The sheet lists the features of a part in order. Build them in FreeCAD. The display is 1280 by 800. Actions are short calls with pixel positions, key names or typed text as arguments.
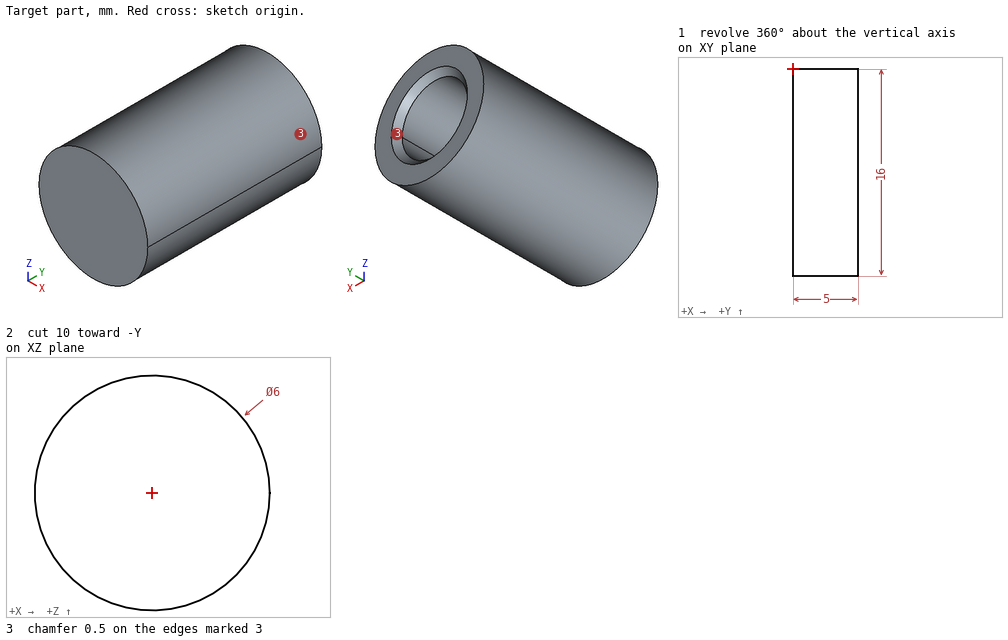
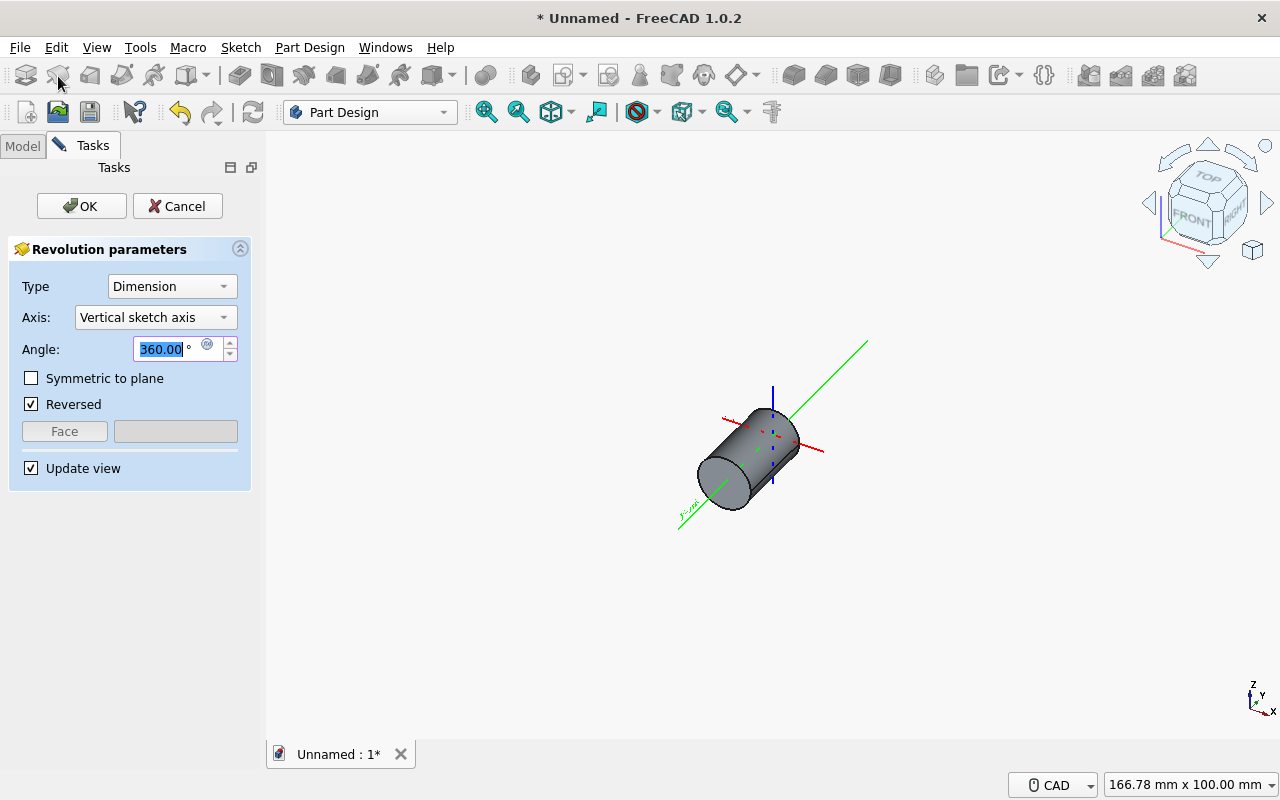
click(82, 206)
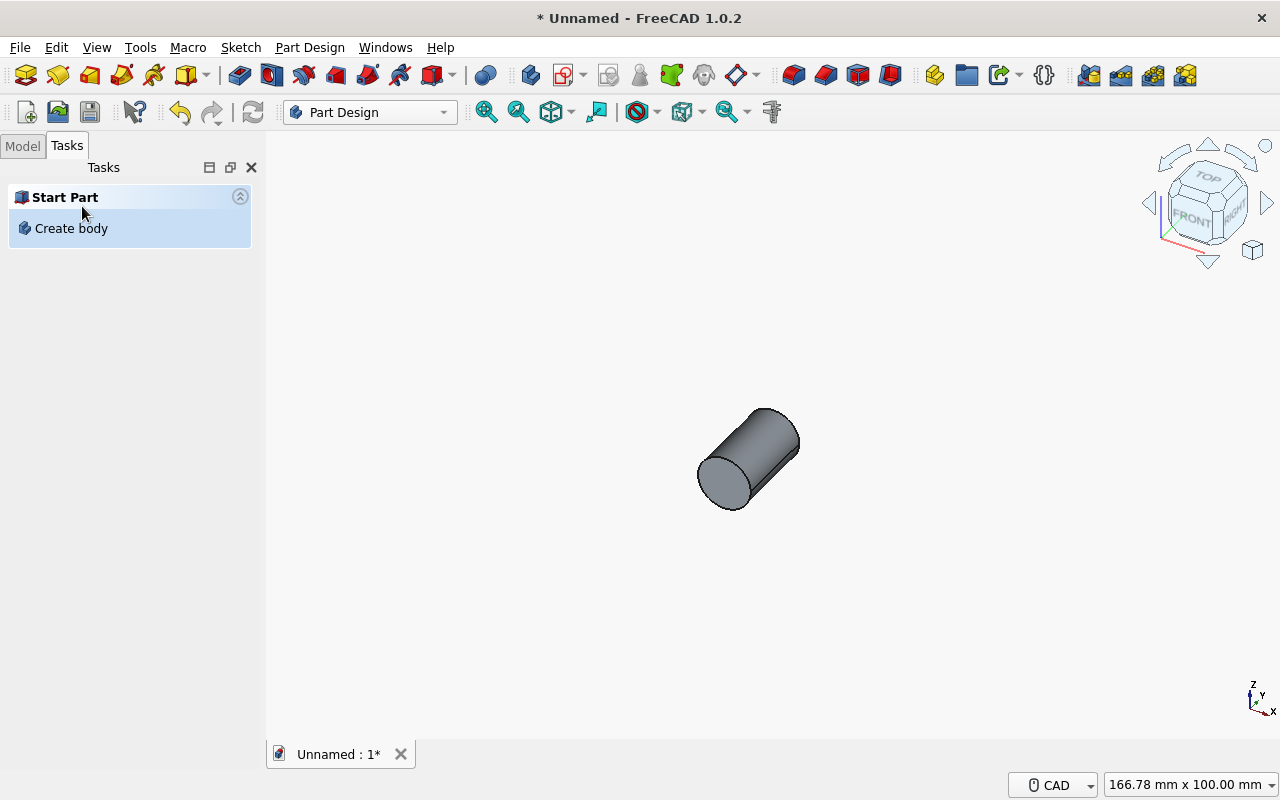
click(488, 112)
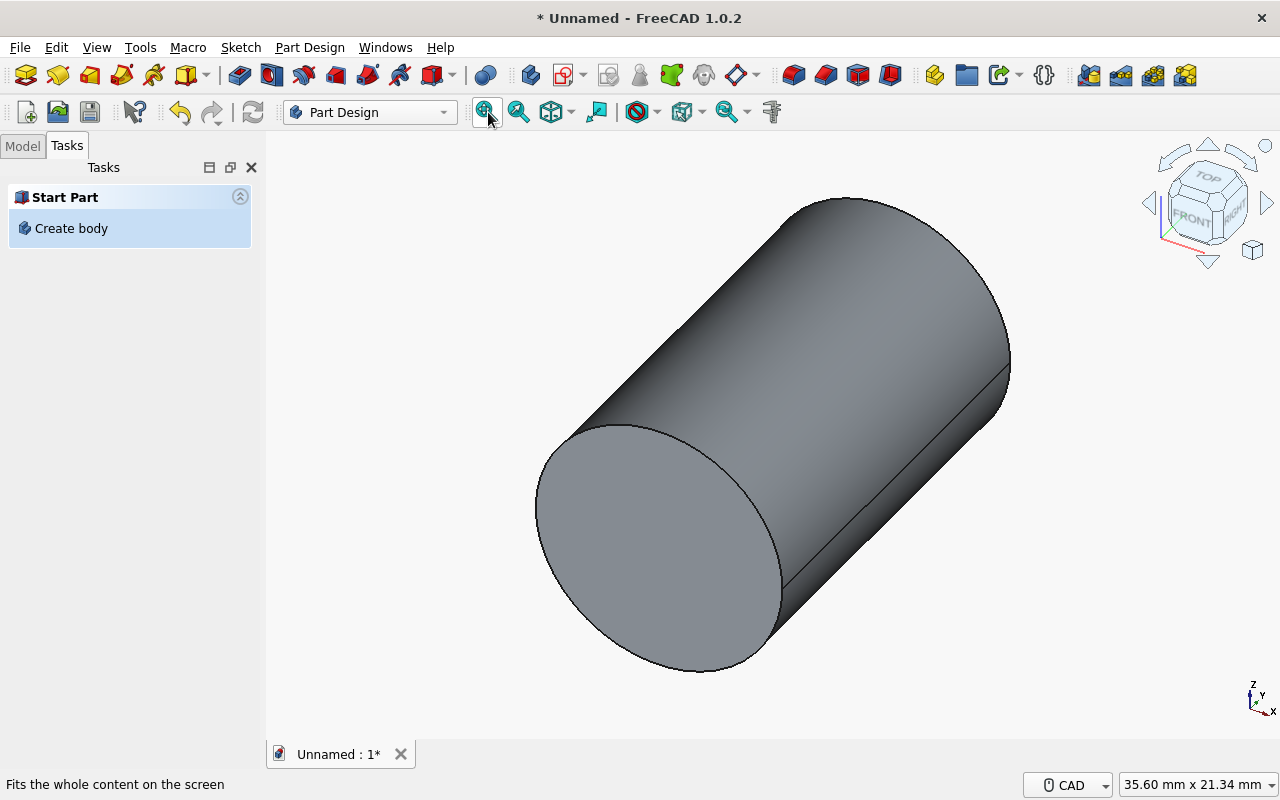
click(564, 76)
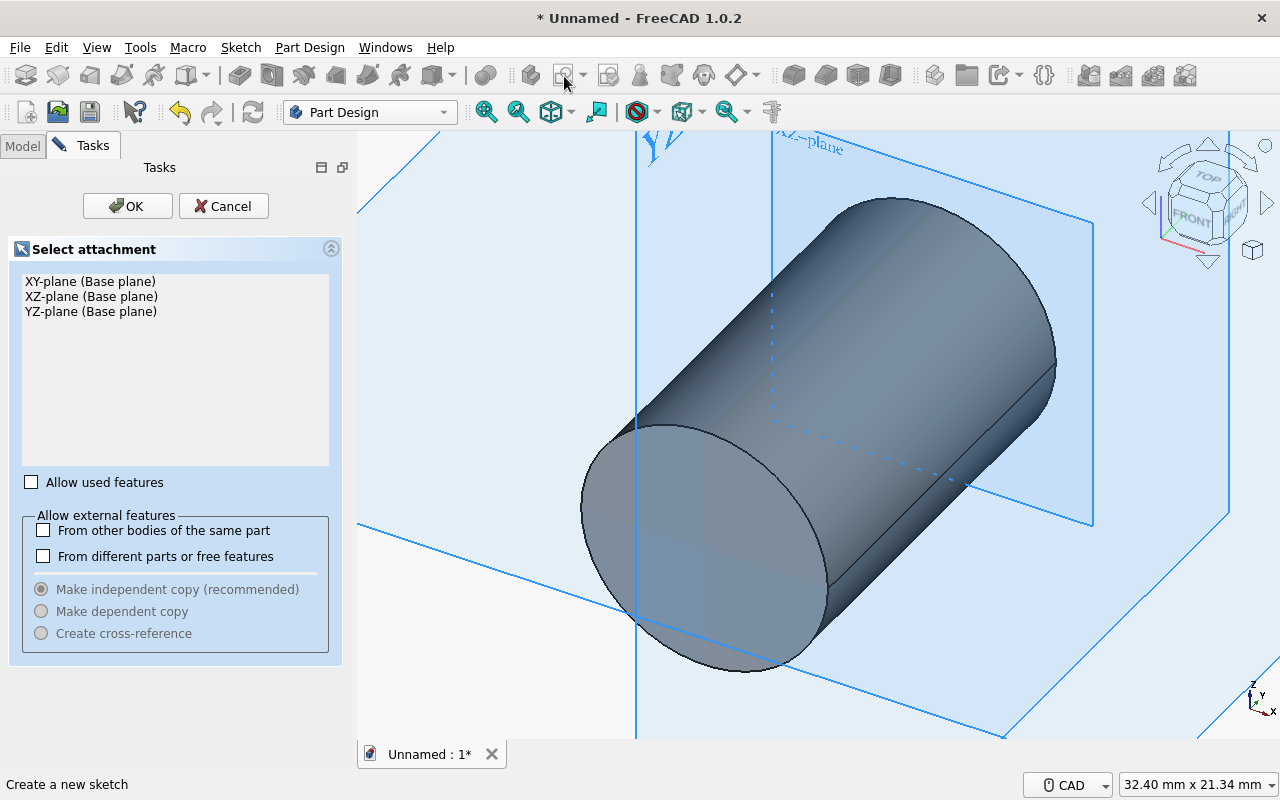
click(82, 296)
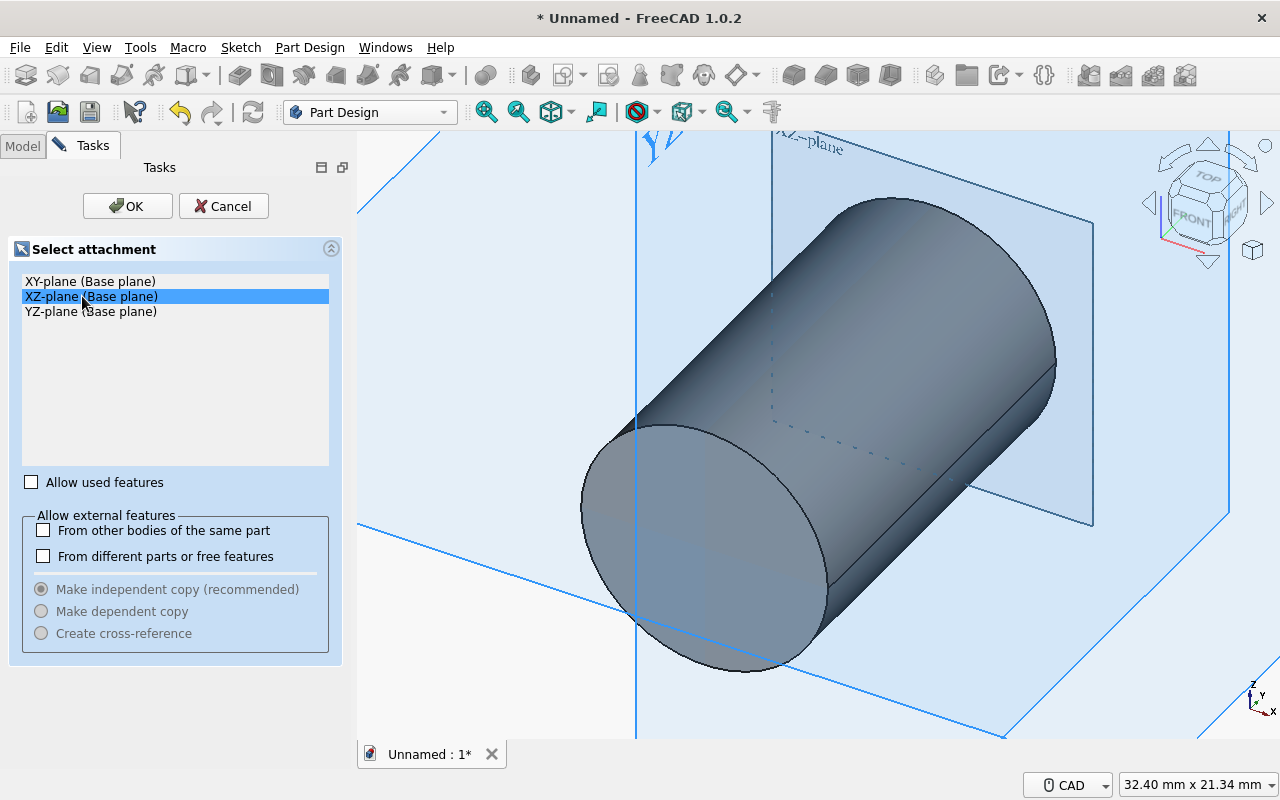
click(128, 206)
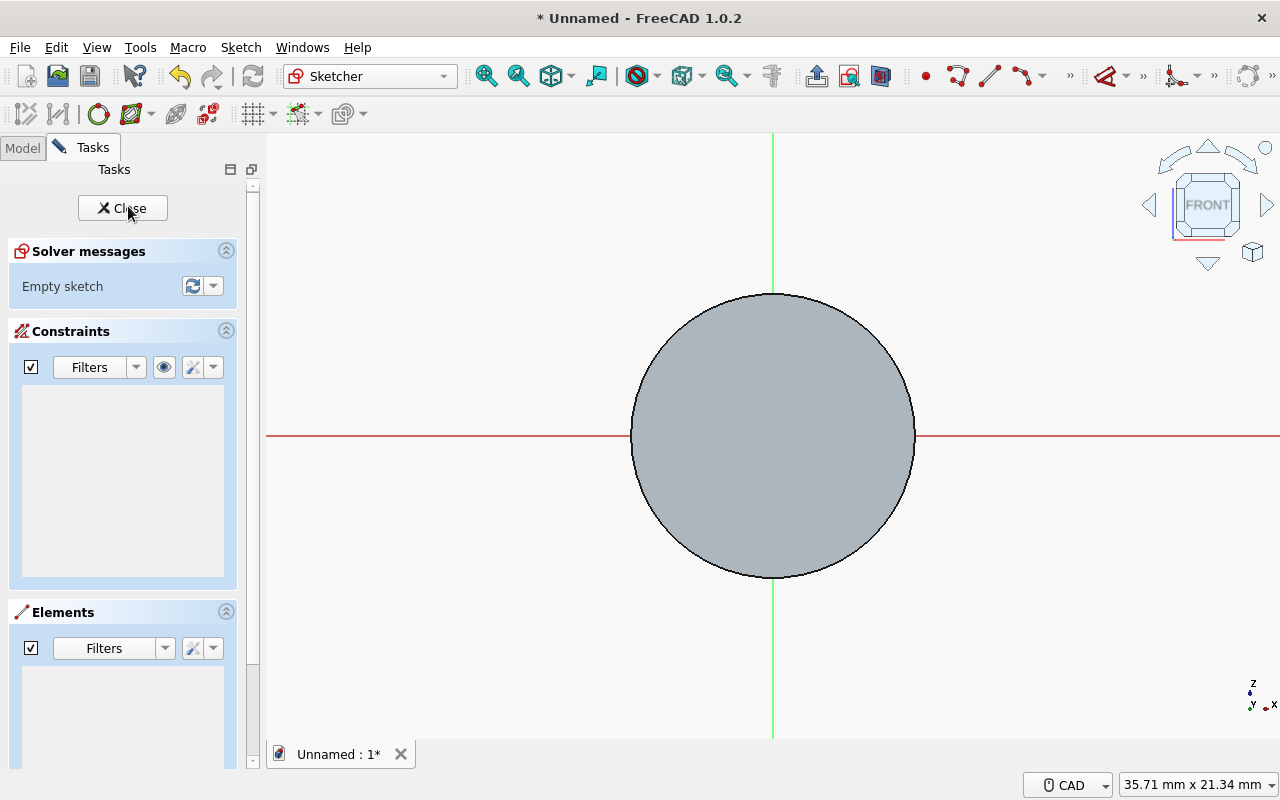
click(882, 76)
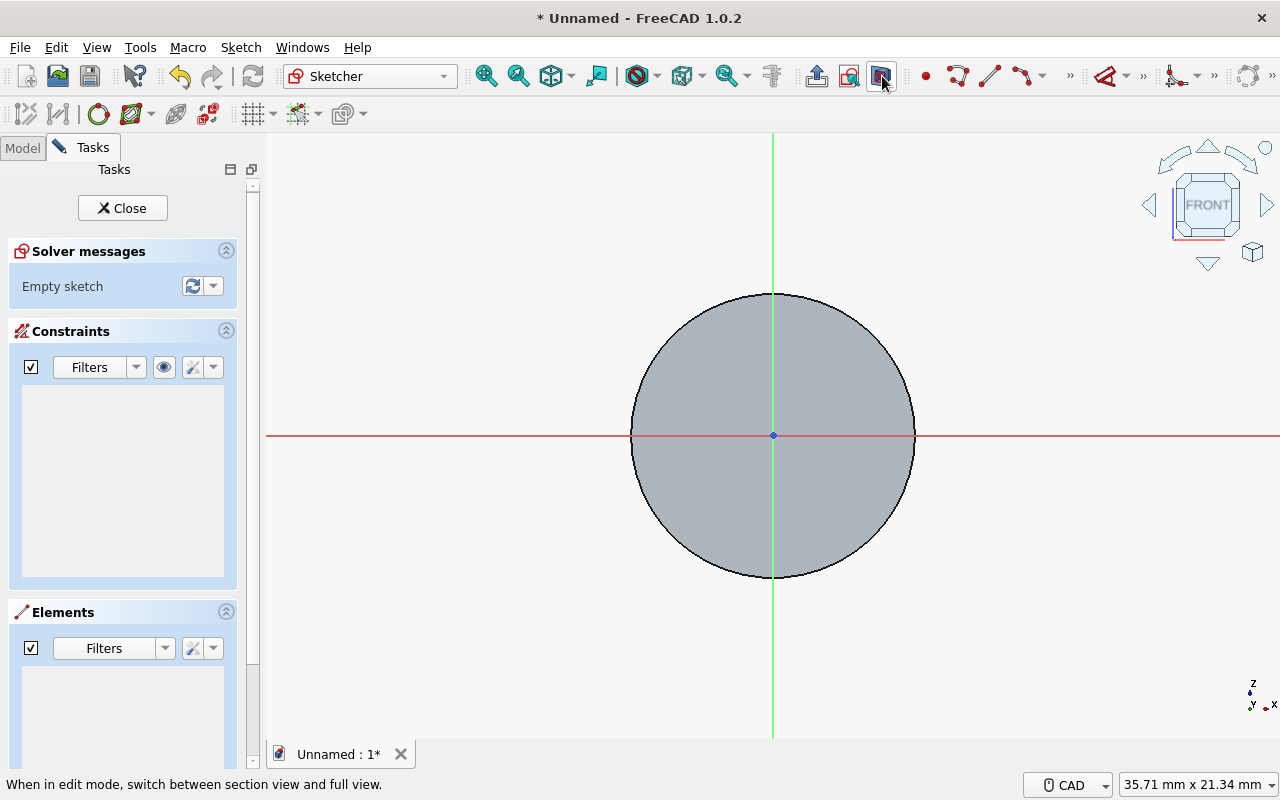
scroll(829, 436, up, 4)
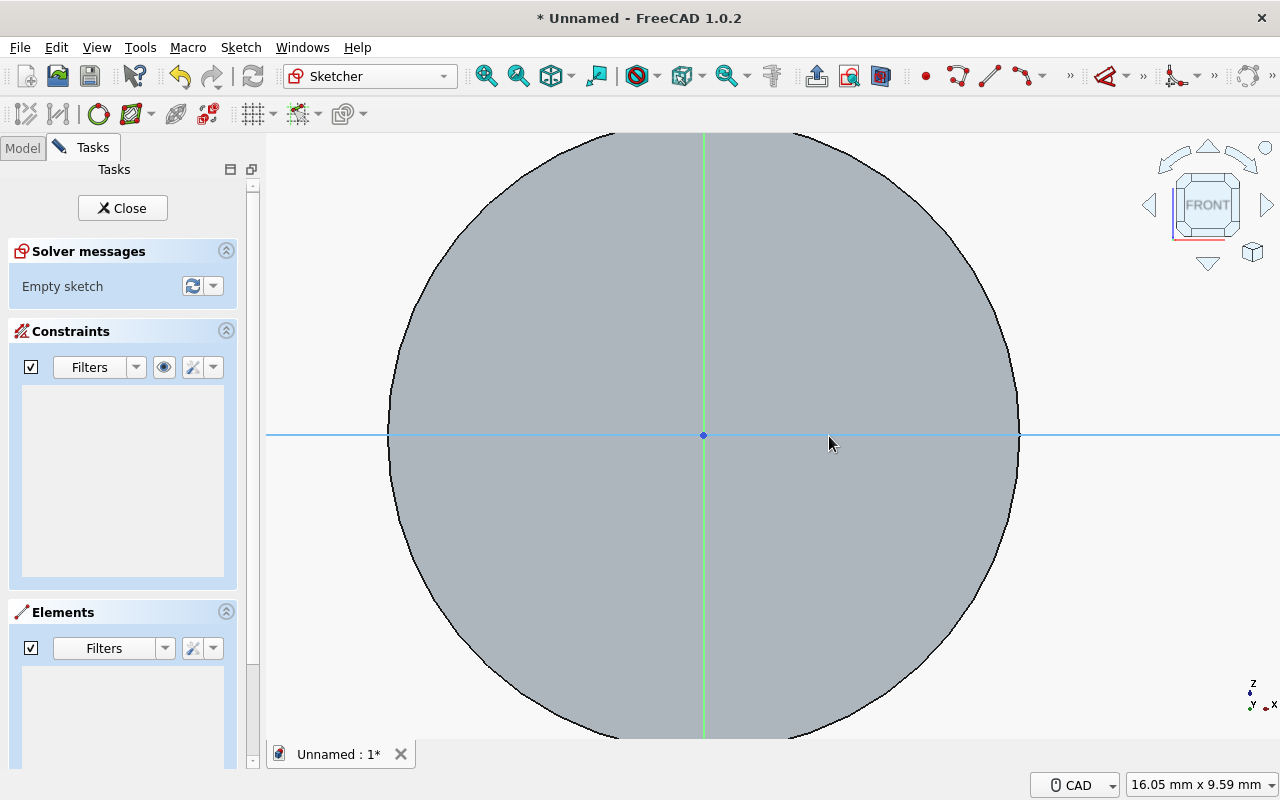
key(g)
key(c)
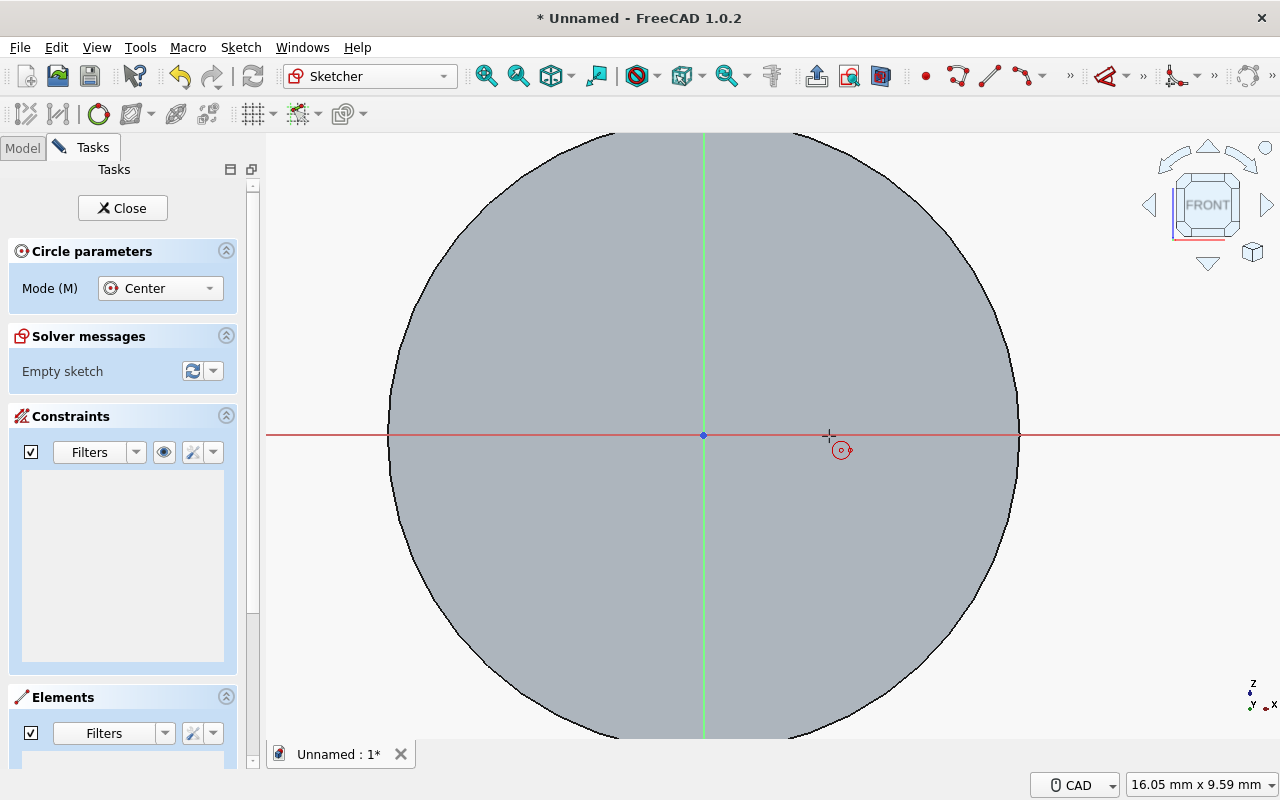
click(704, 435)
move(838, 301)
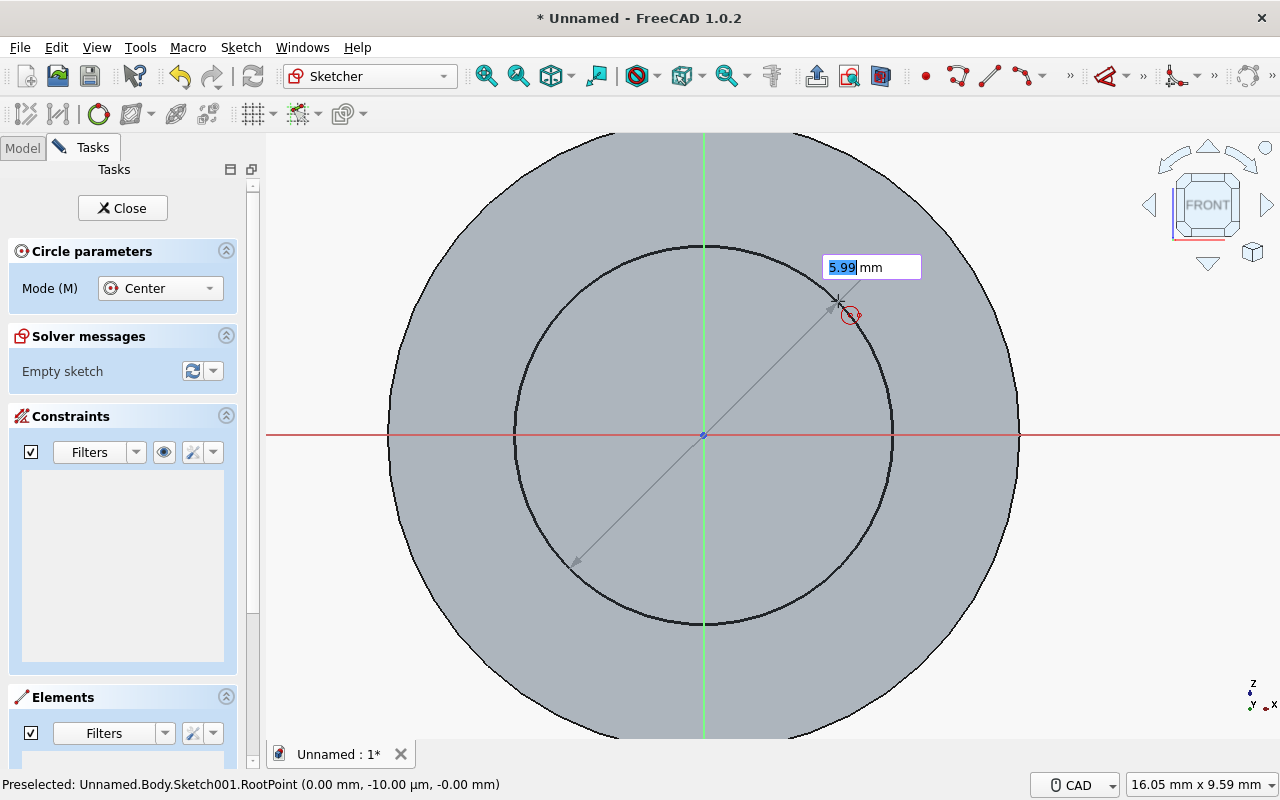
text(6)
key(Return)
key(Escape)